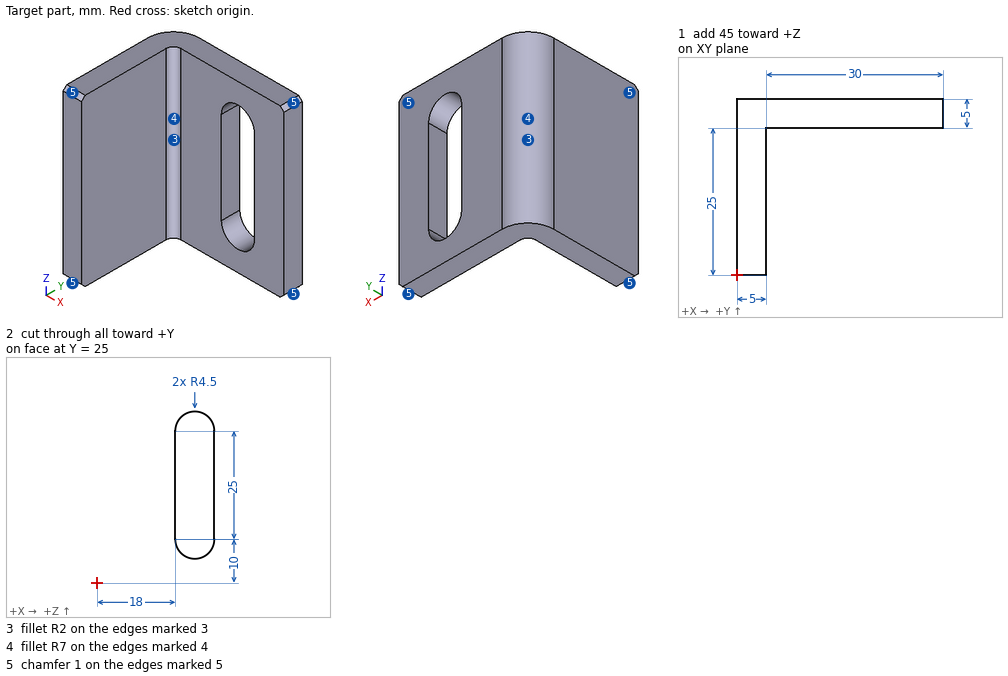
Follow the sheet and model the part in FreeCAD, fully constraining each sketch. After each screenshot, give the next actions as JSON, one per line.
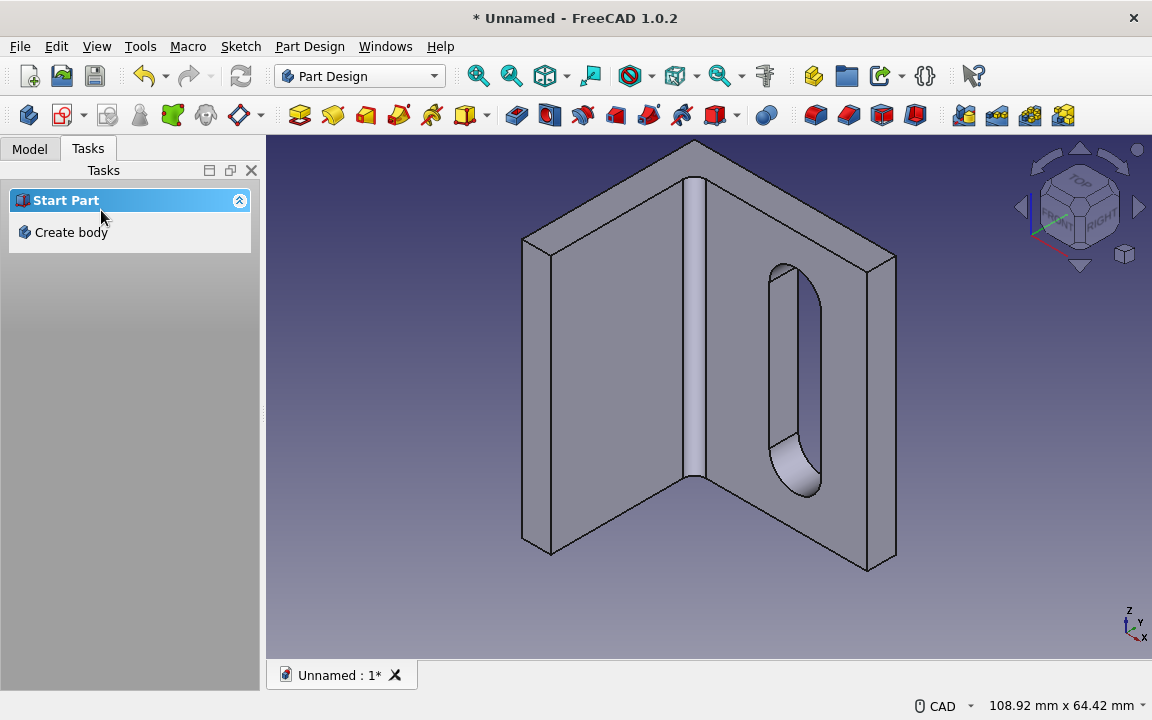
{"action": "key", "text": "1"}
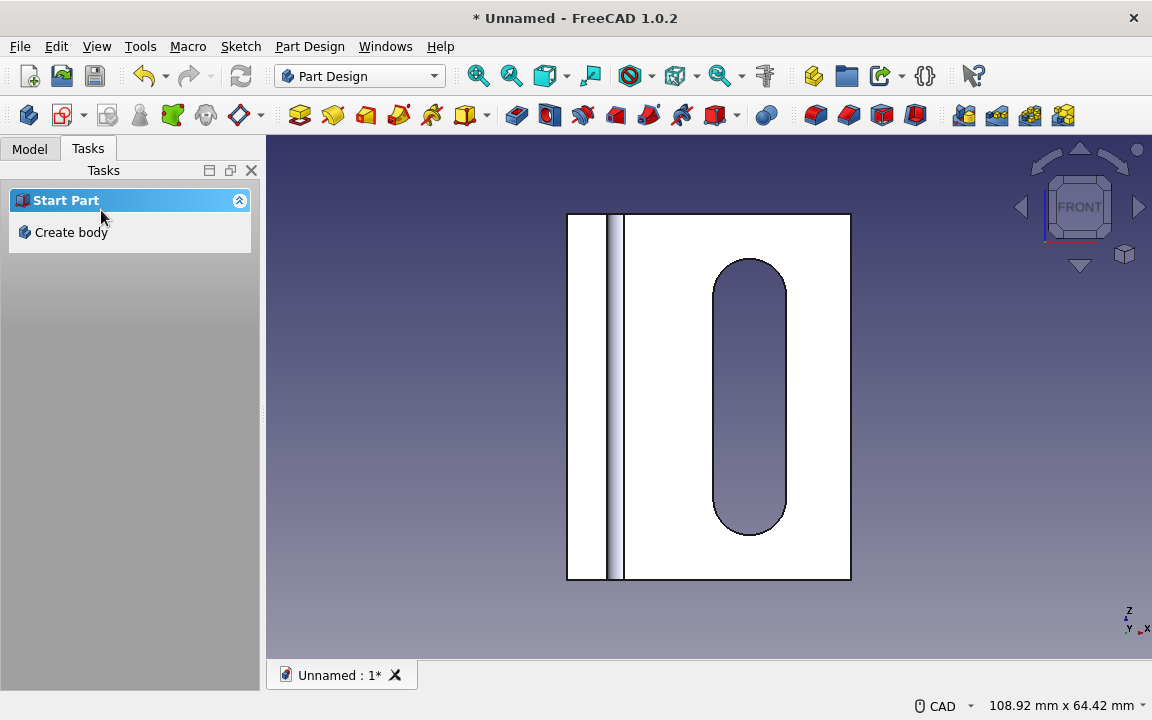
{"action": "key", "text": "3"}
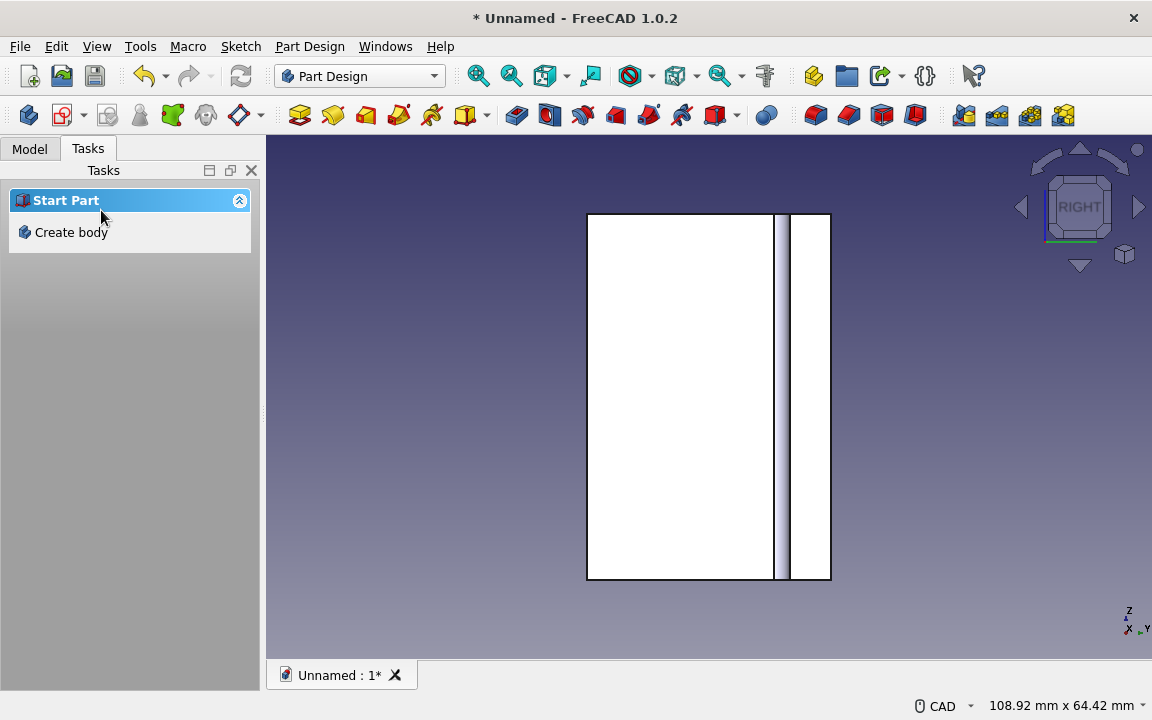
{"action": "key", "text": "5"}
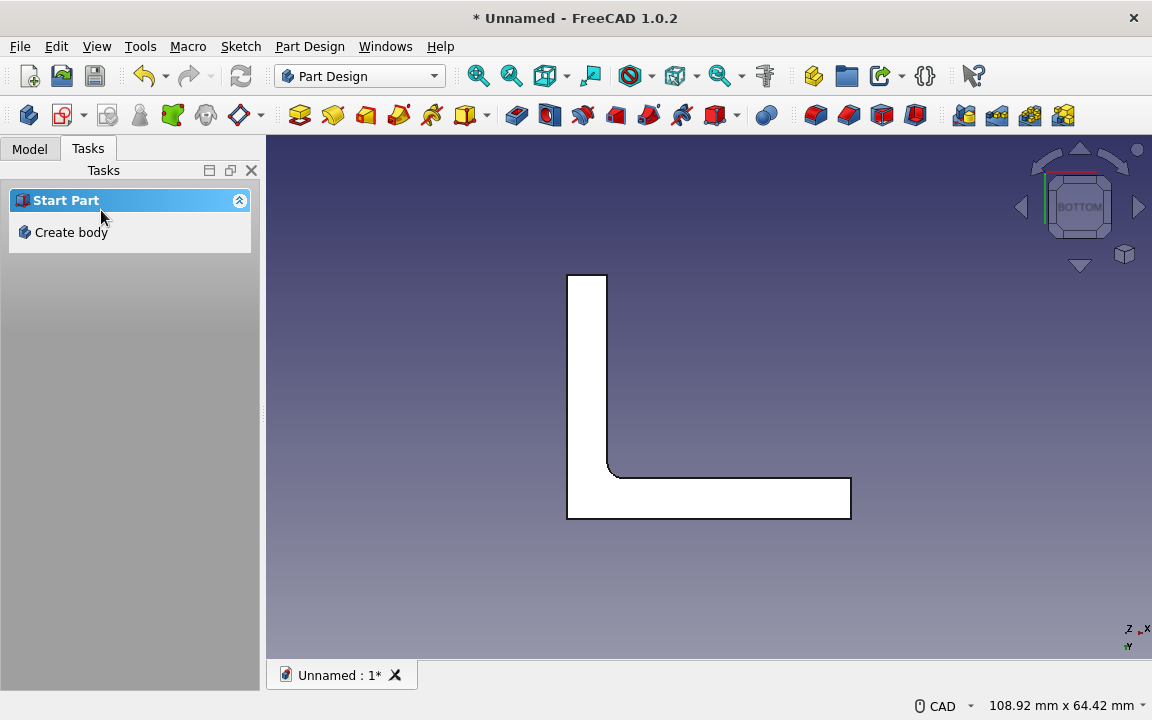
{"action": "key", "text": "4"}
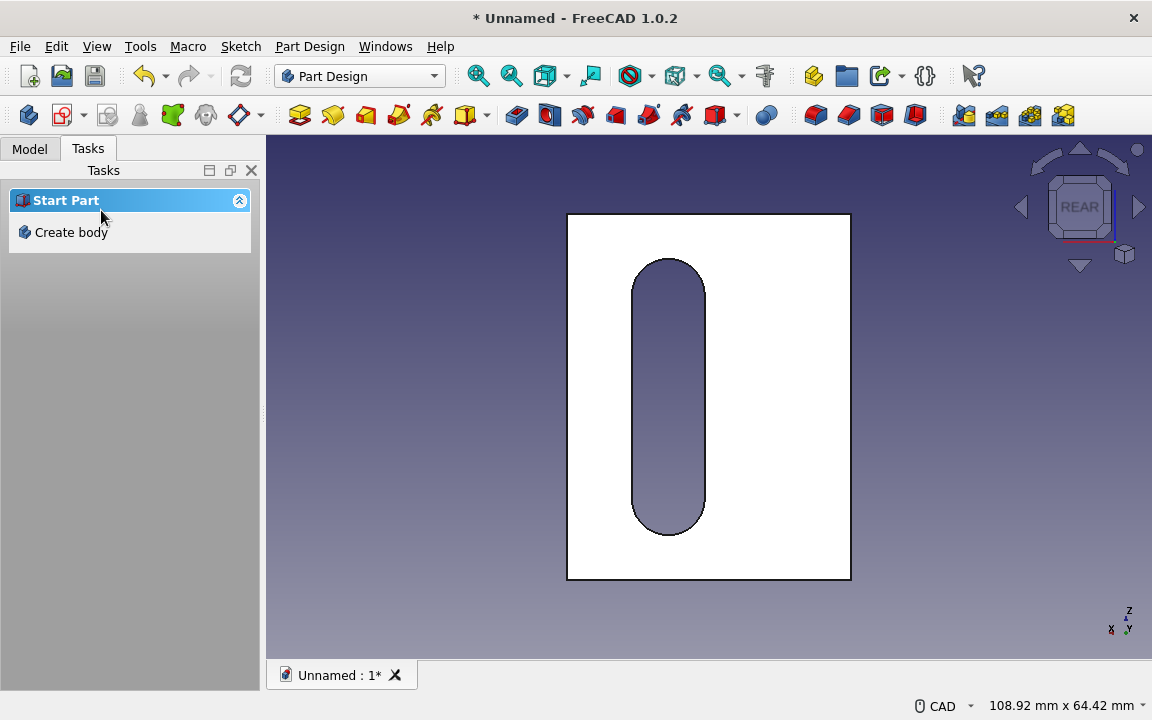
{"action": "left_click", "coordinate": [851, 396]}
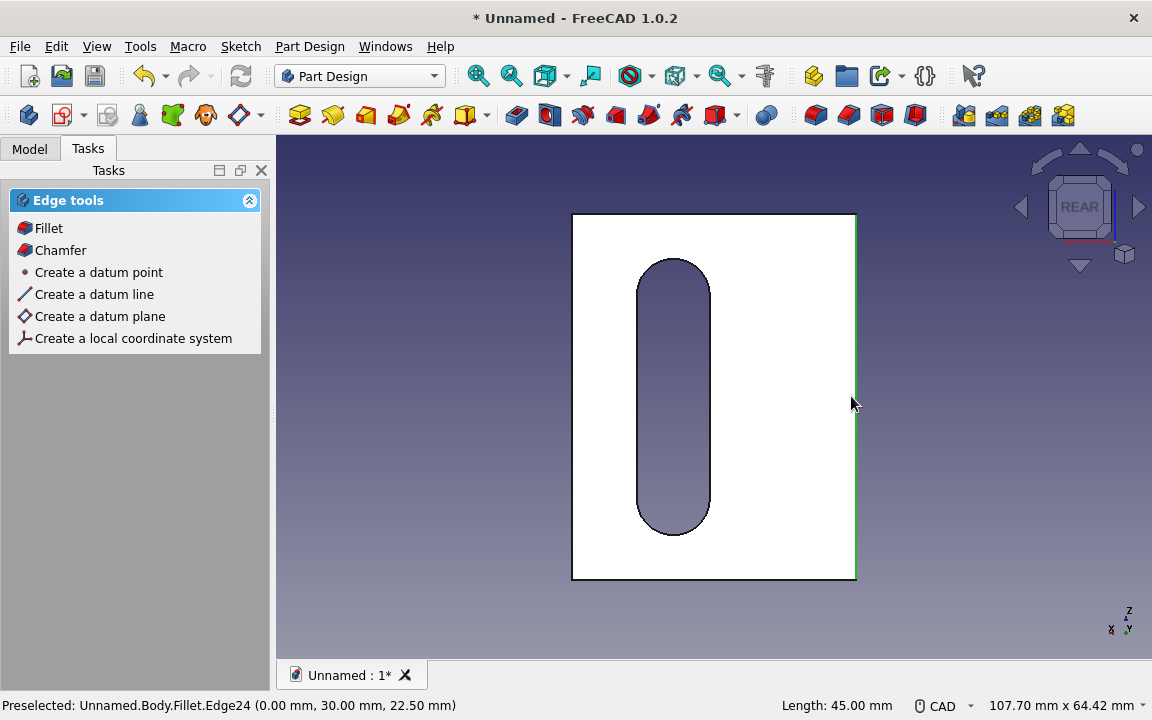
{"action": "left_click", "coordinate": [816, 116]}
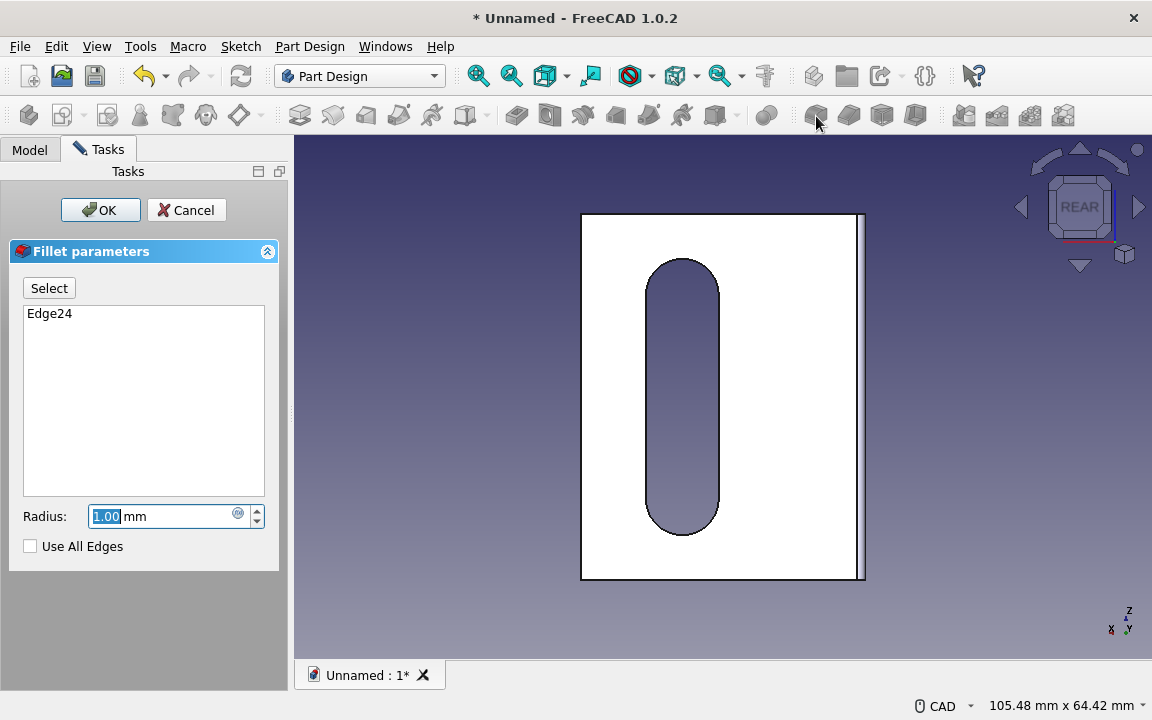
{"action": "type", "text": "7"}
{"action": "key", "text": "Tab"}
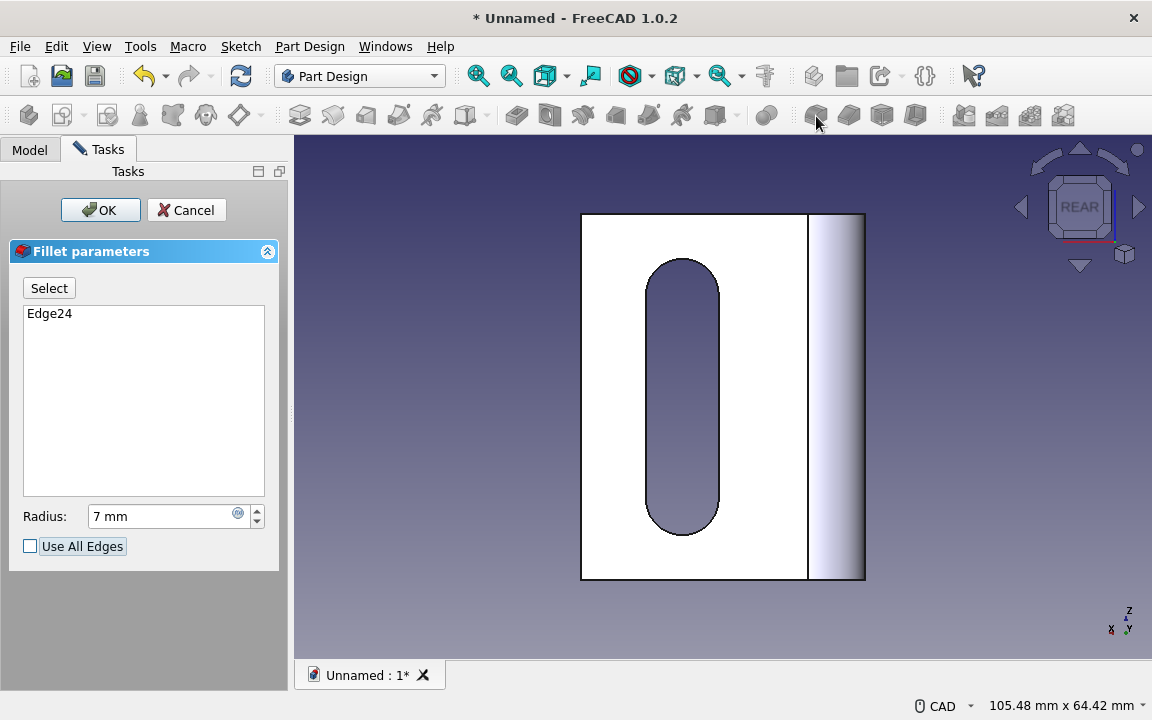
{"action": "left_click", "coordinate": [101, 210]}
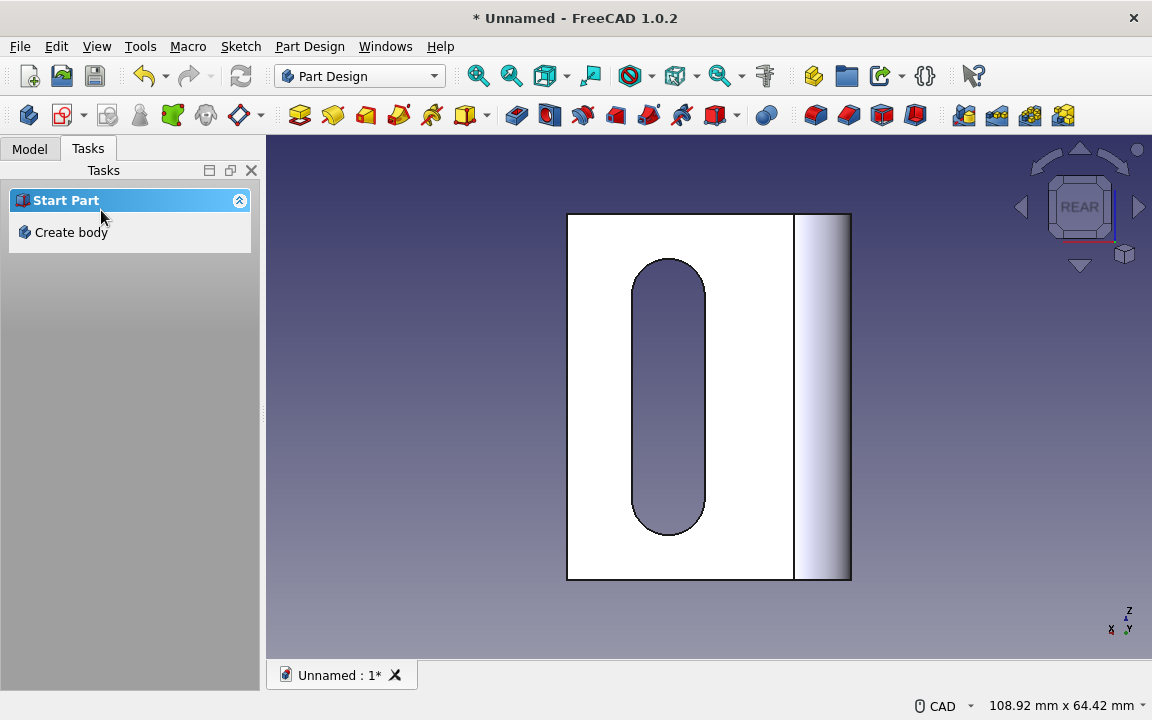
{"action": "key", "text": "0"}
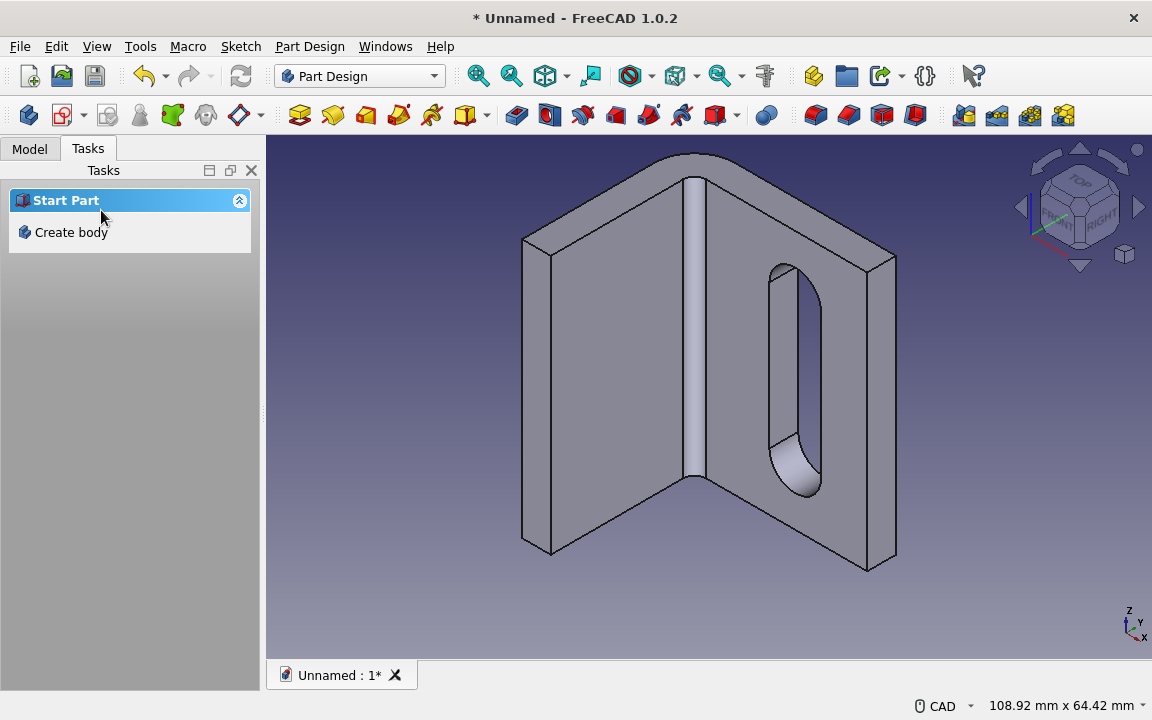
{"action": "left_click", "coordinate": [536, 247]}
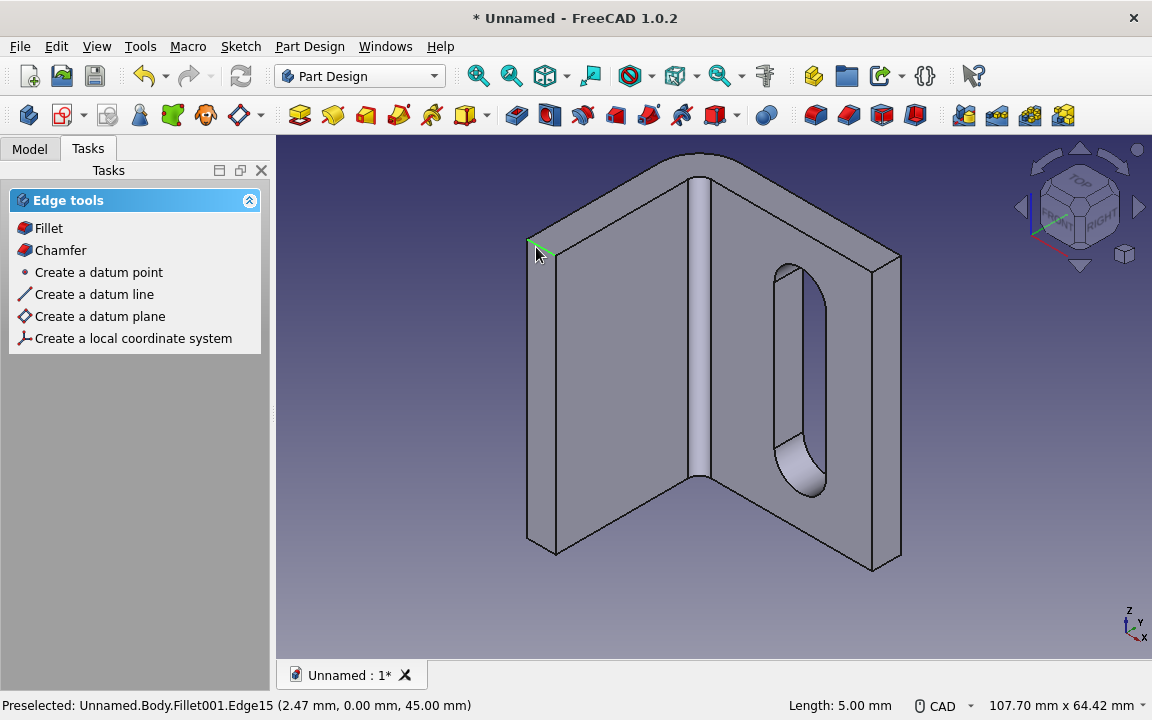
{"action": "left_click", "coordinate": [887, 263], "text": "ctrl"}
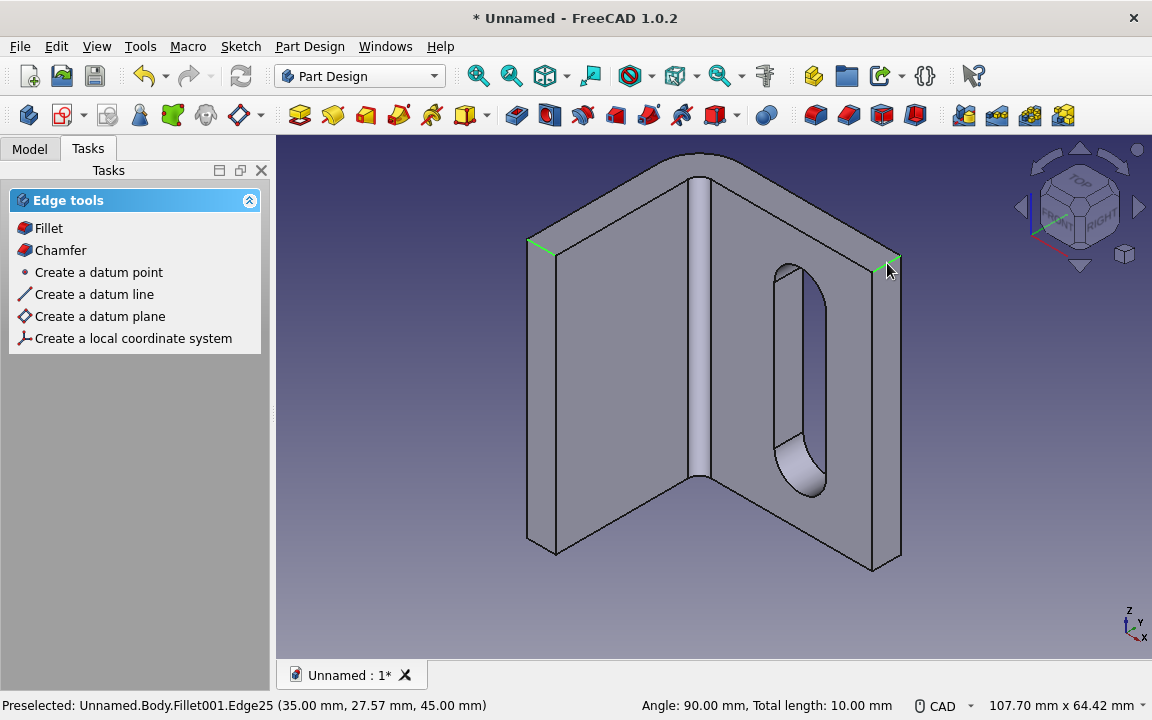
{"action": "key", "text": "2"}